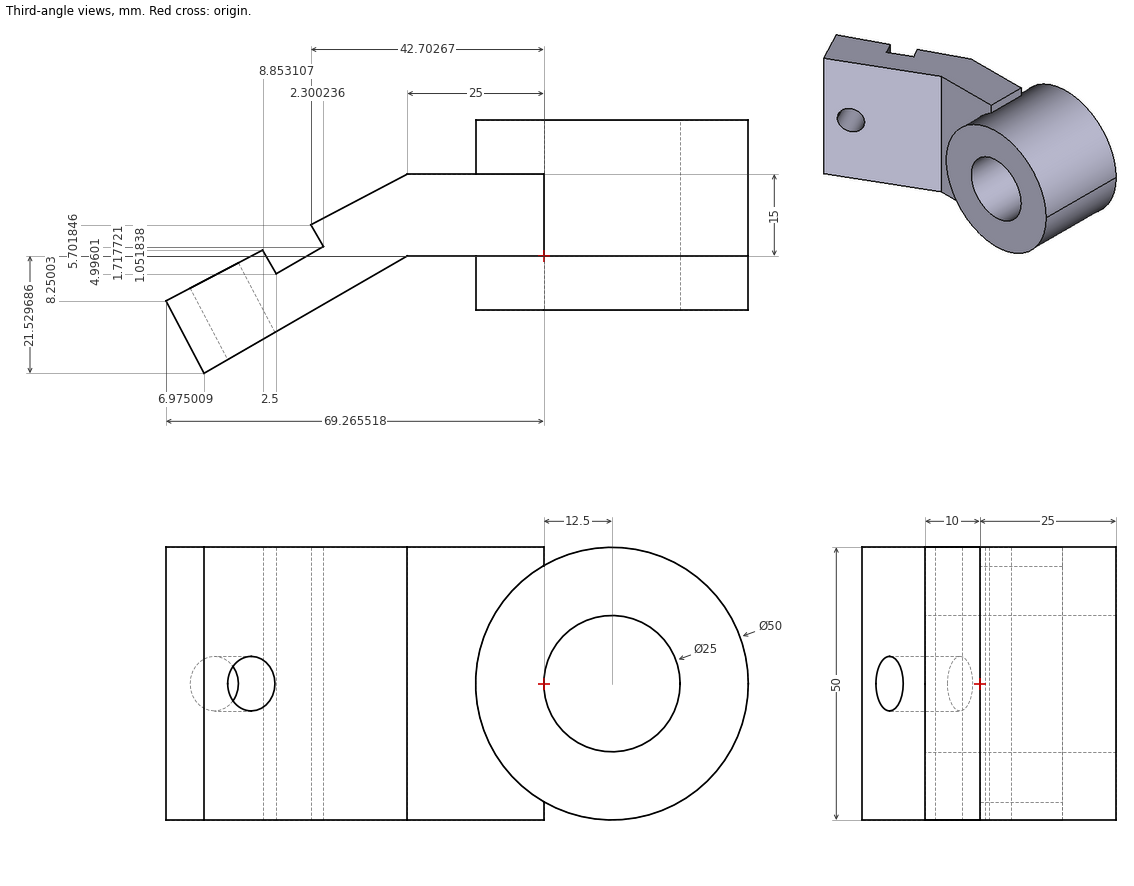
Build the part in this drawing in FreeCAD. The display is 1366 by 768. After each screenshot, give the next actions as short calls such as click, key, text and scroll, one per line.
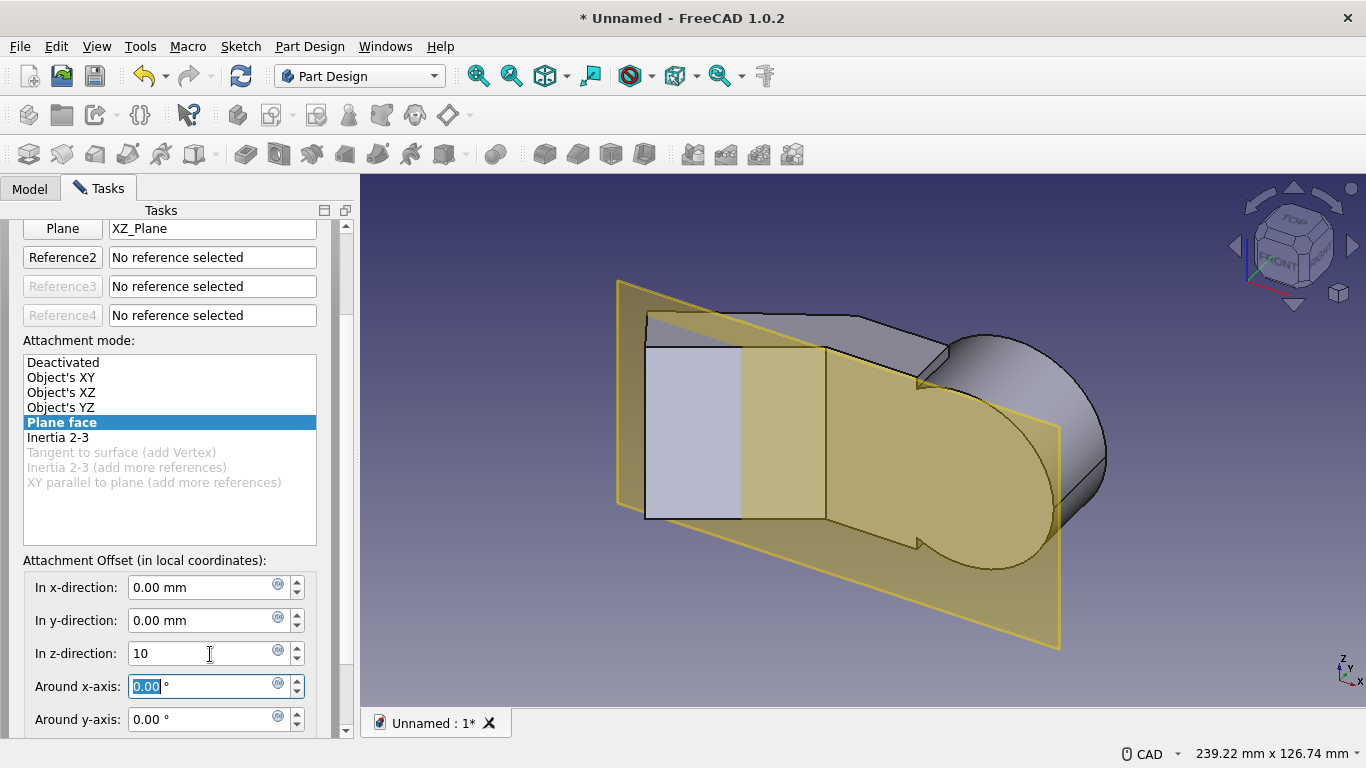
scroll(346, 479, up, 3)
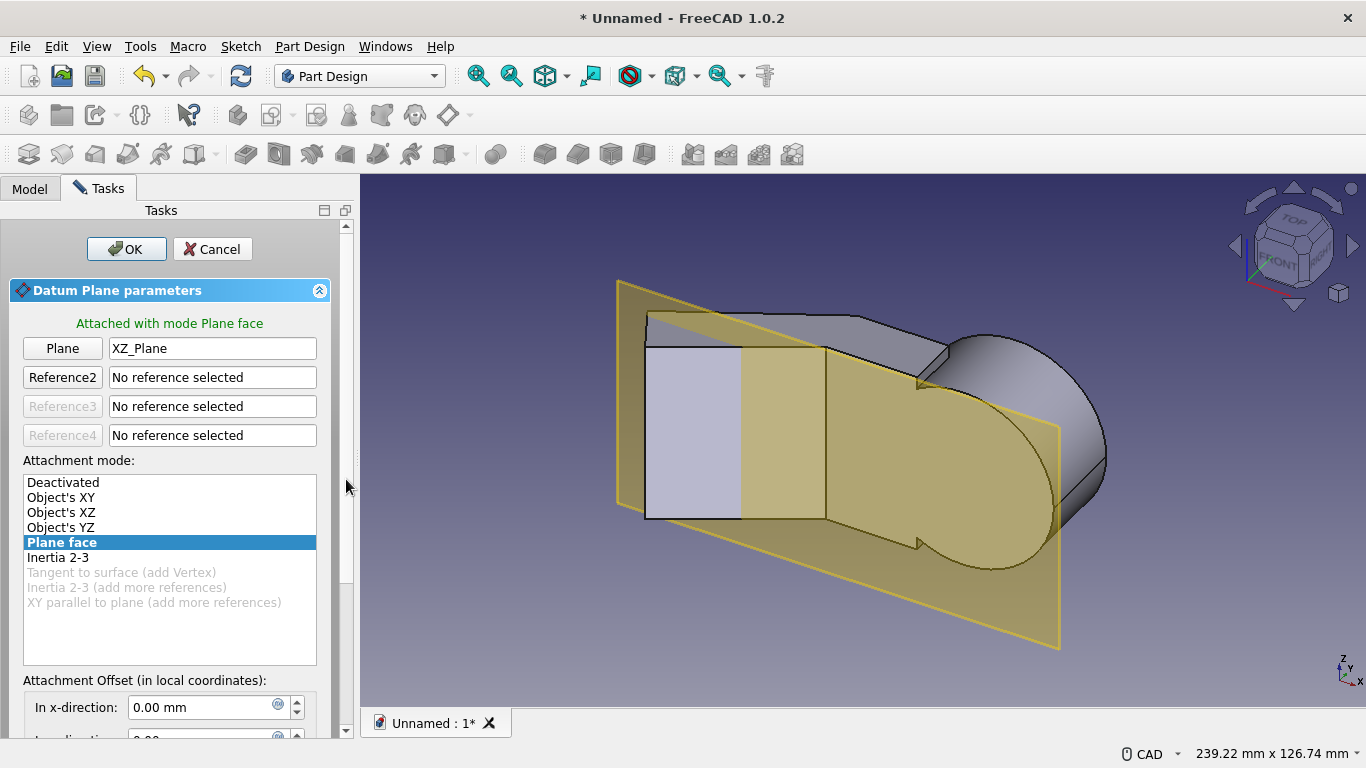
click(127, 249)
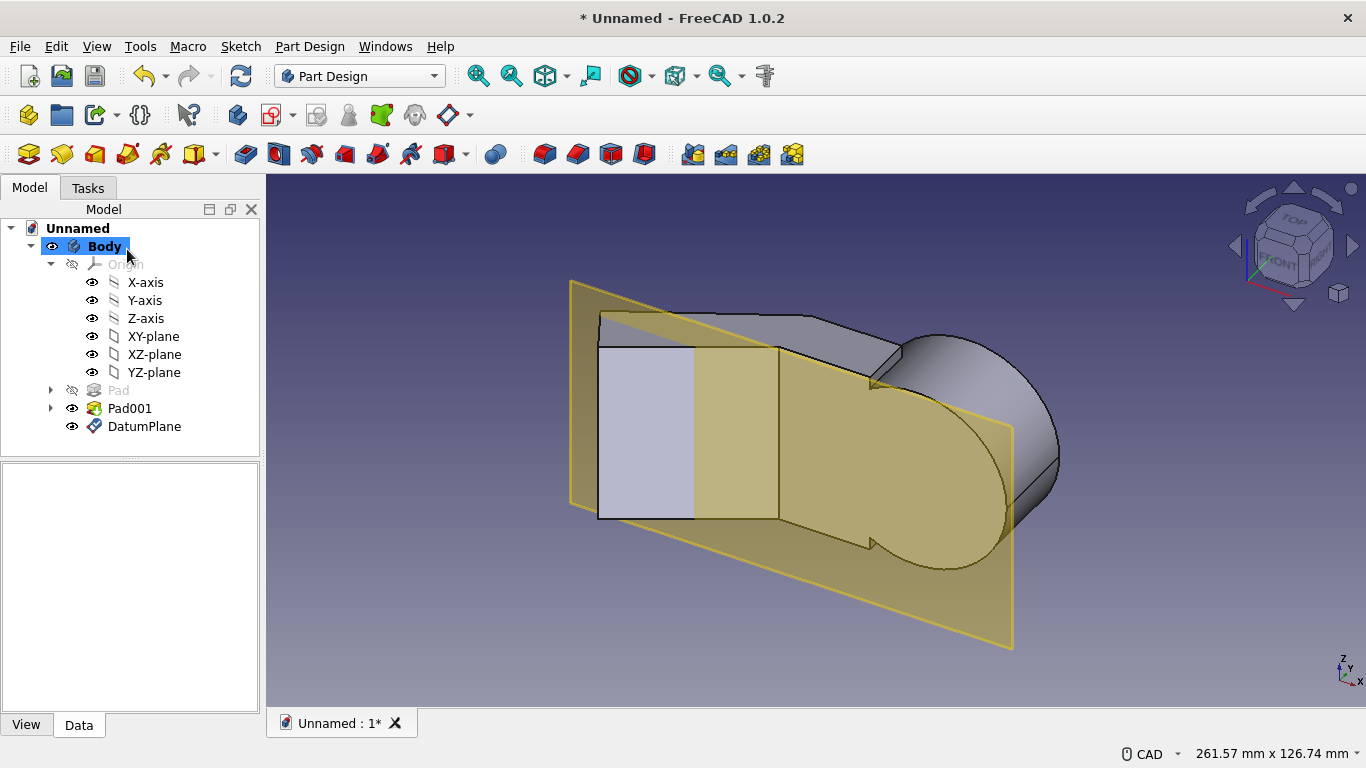
click(117, 426)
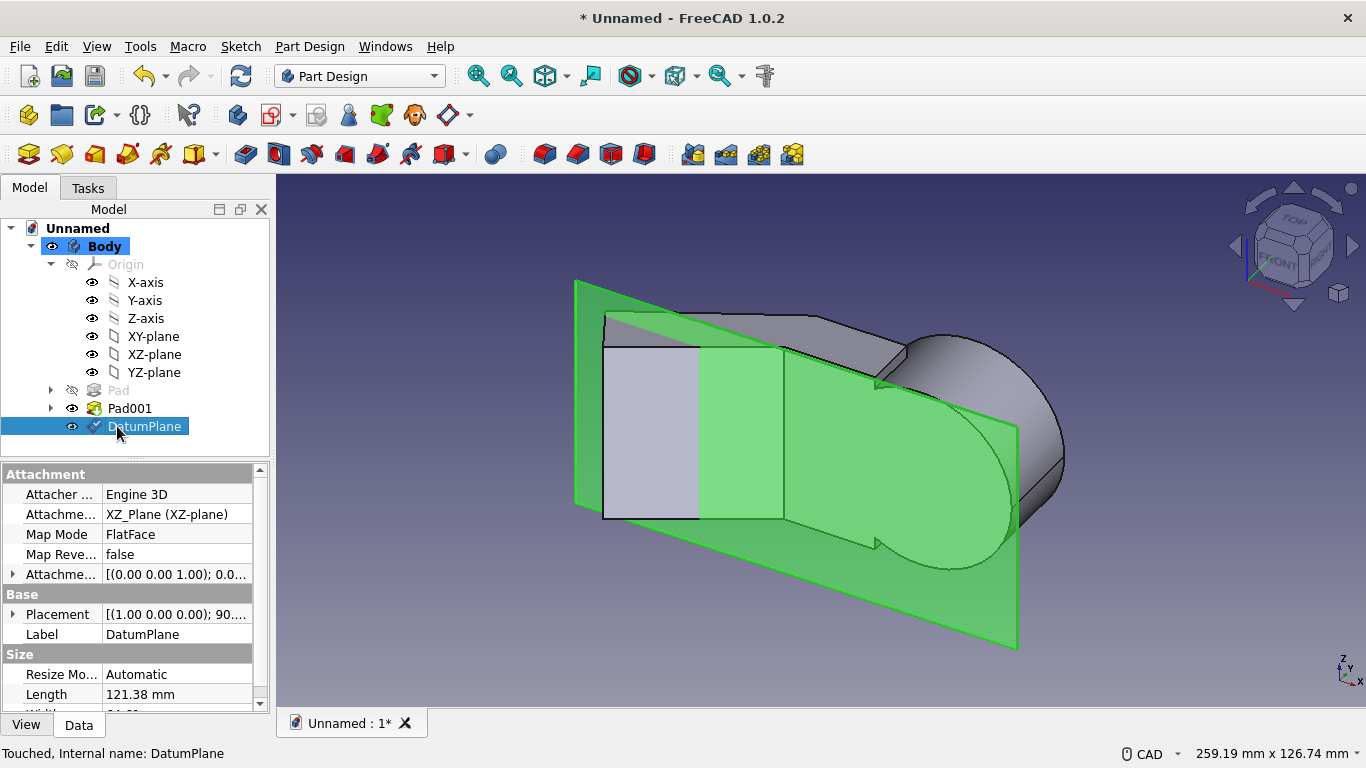
click(270, 116)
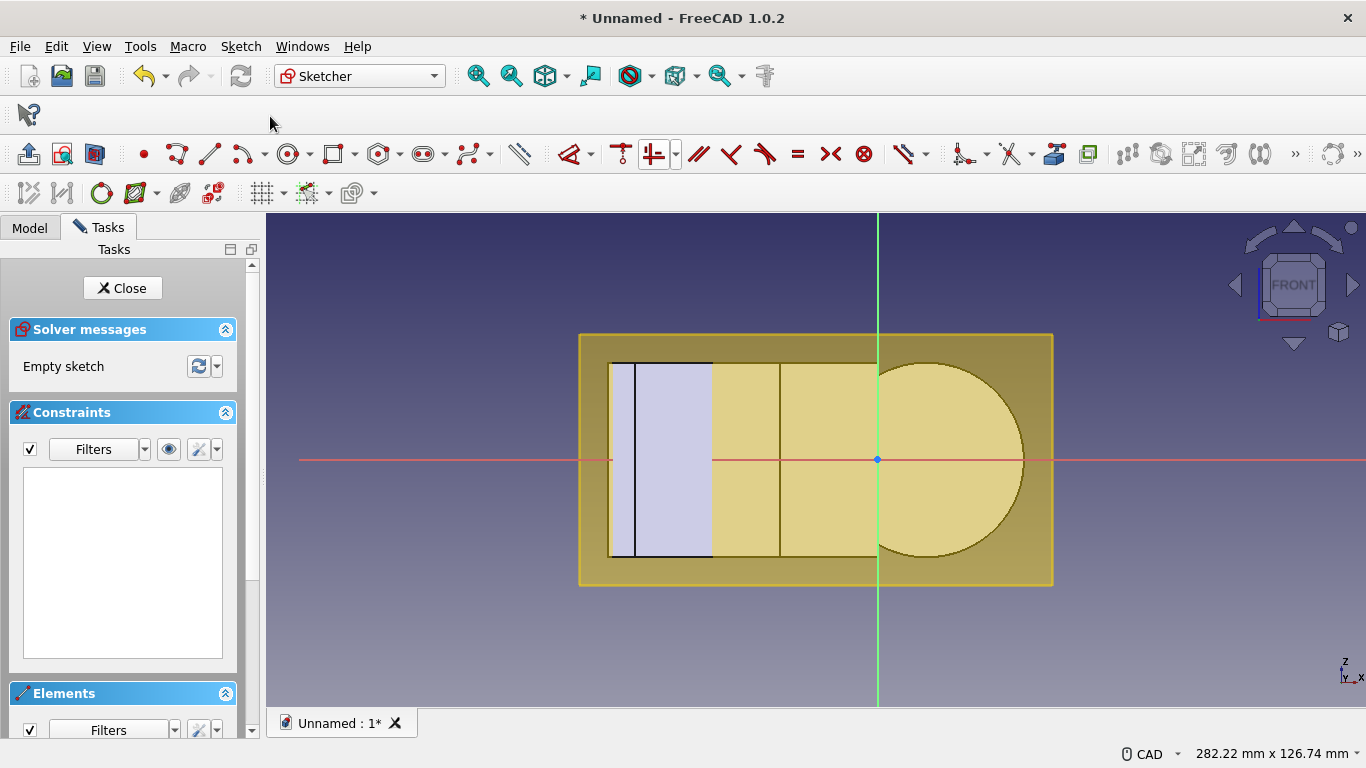
key(q)
key(s)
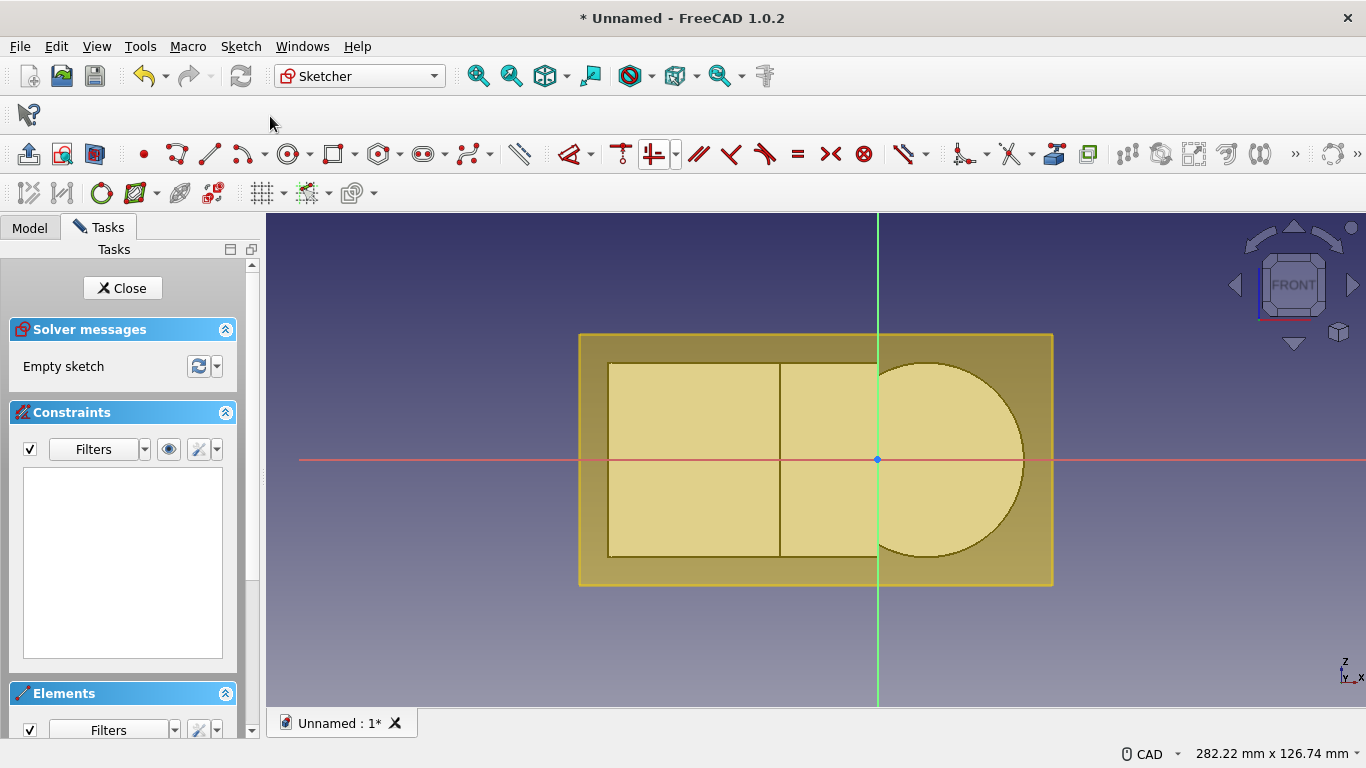
scroll(1201, 460, up, 2)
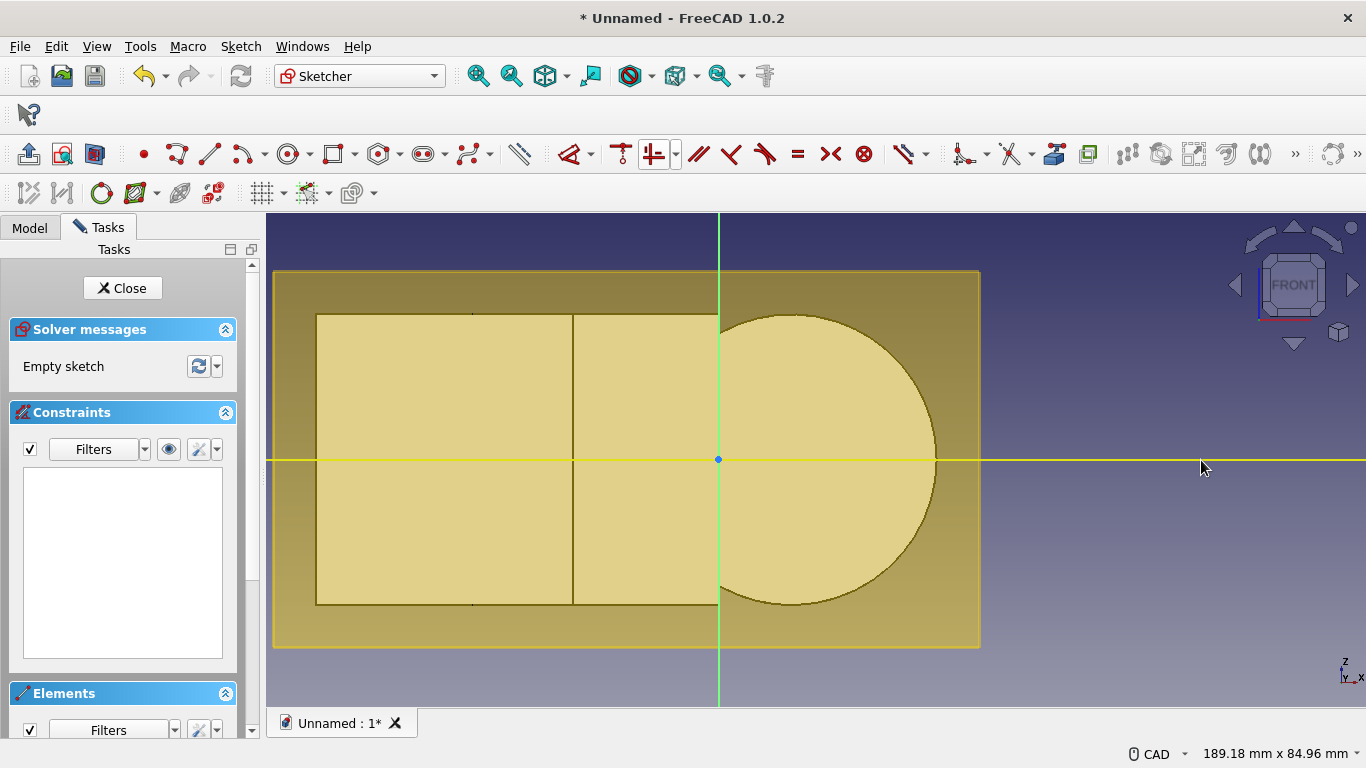
key(g)
key(c)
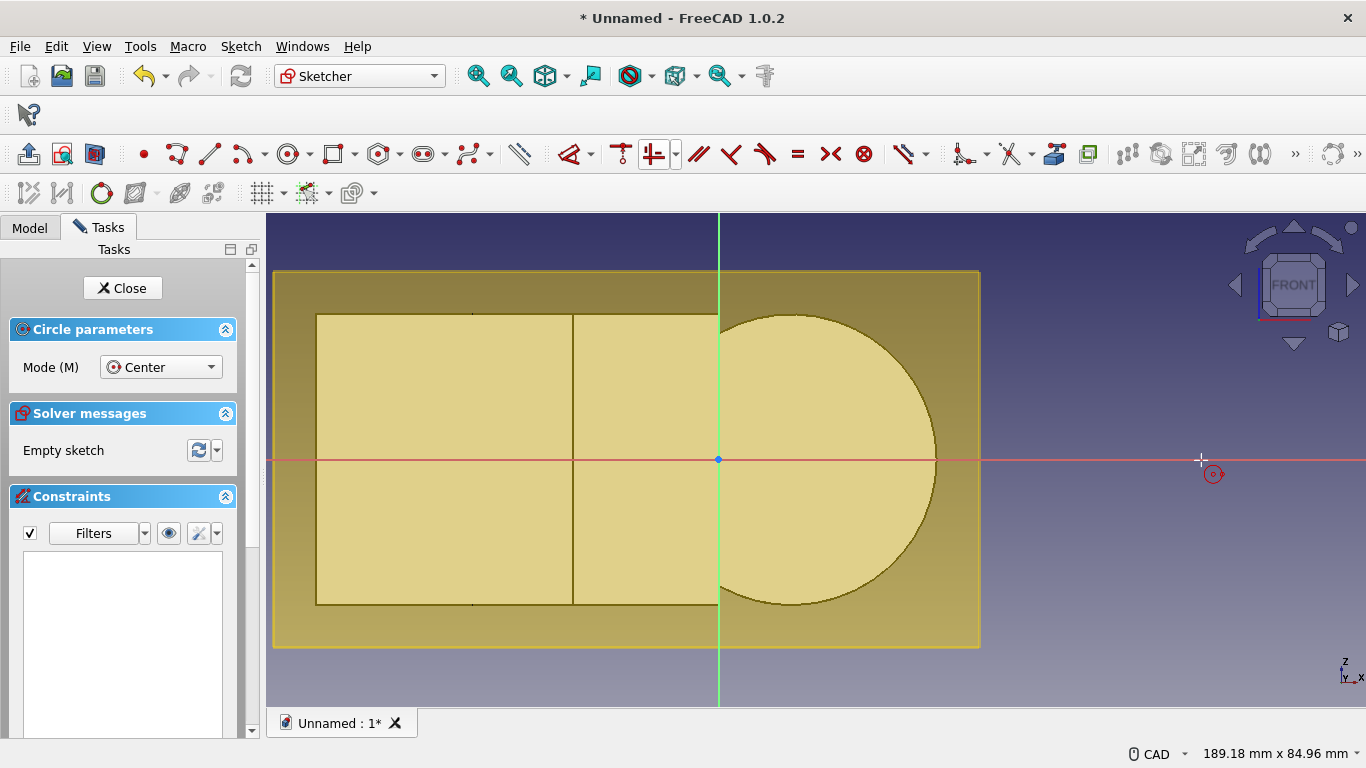
click(791, 460)
click(894, 357)
key(Escape)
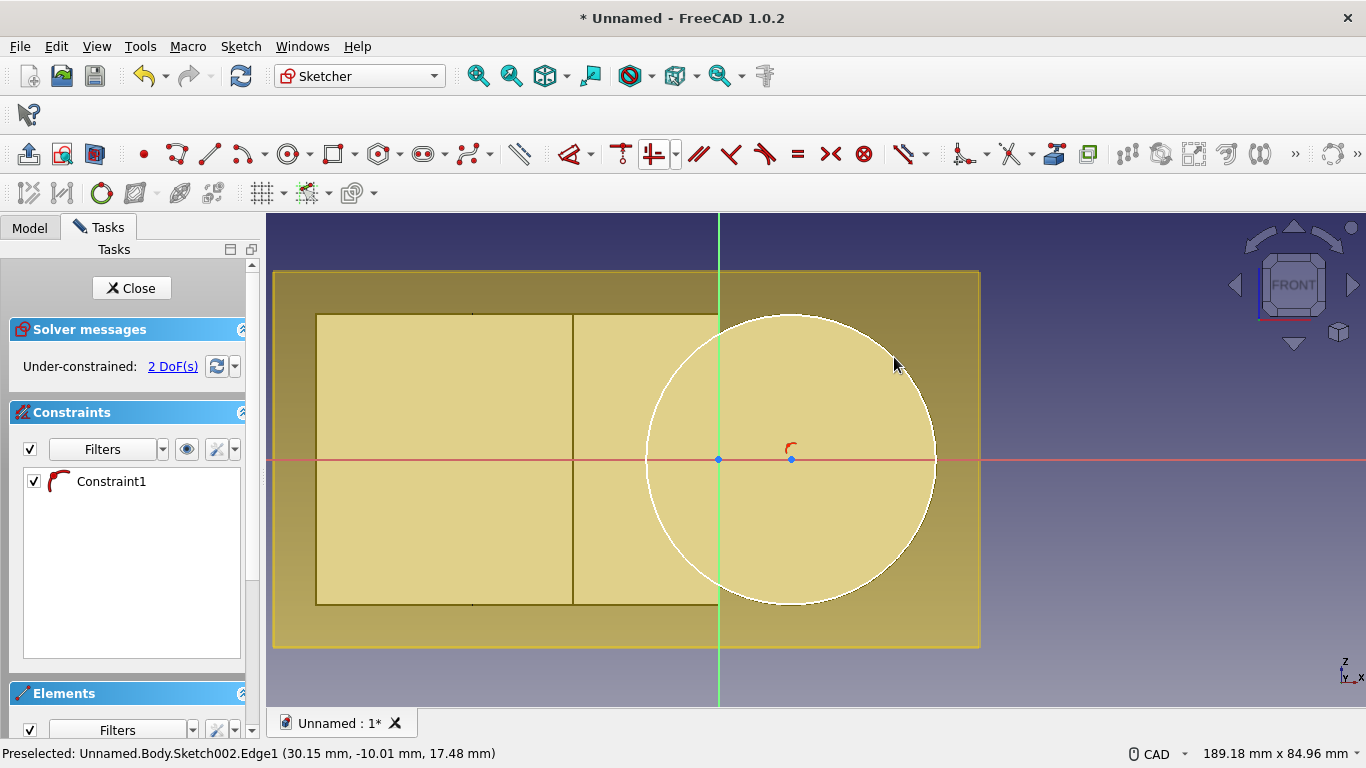
key(d)